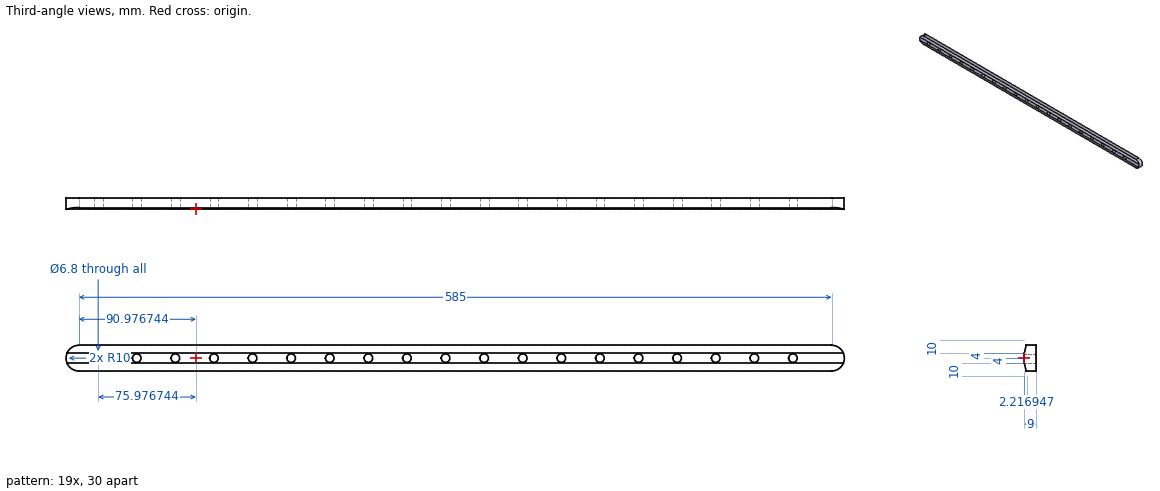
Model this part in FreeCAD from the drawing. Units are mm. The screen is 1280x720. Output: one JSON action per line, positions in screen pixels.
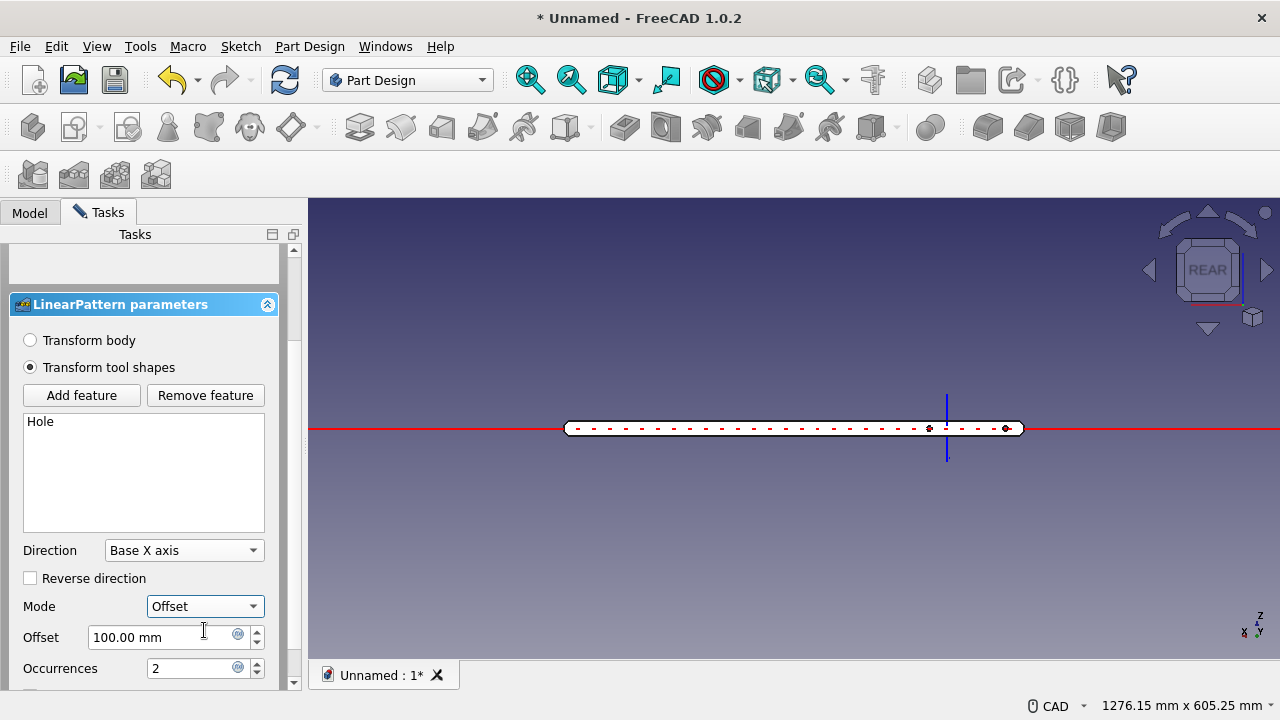
{"action": "triple_click", "coordinate": [170, 638]}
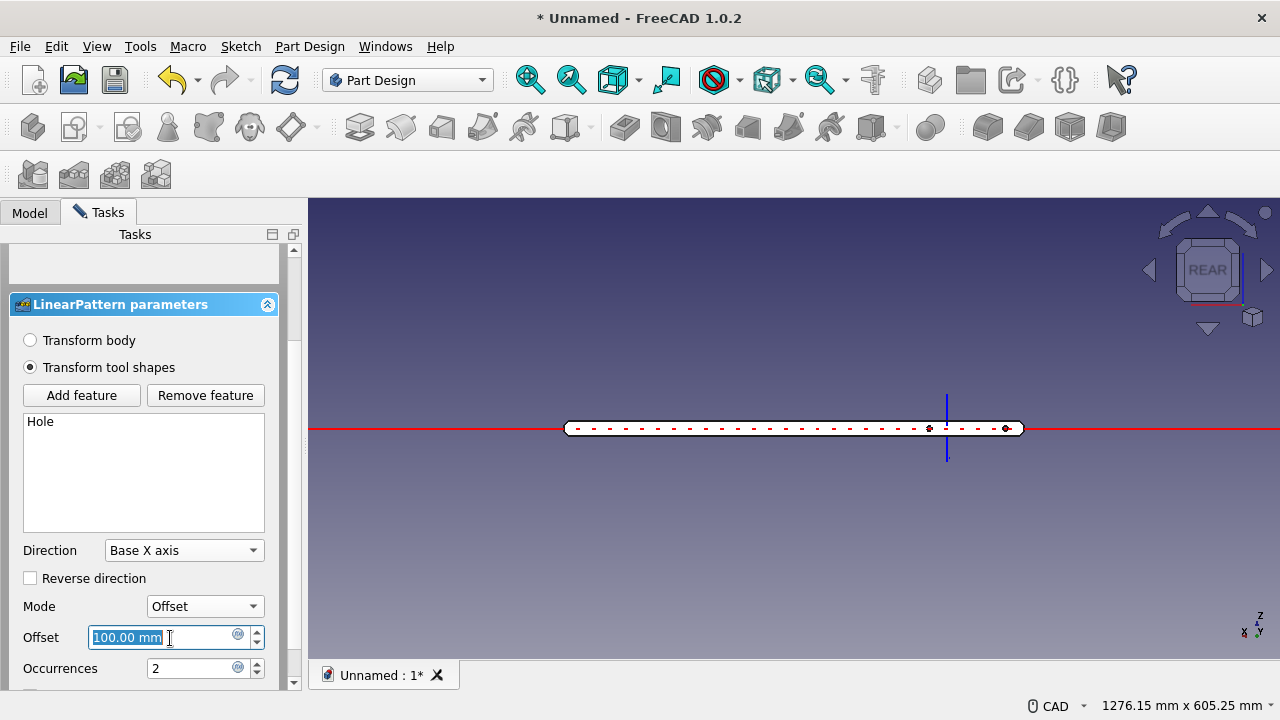
{"action": "type", "text": "30"}
{"action": "key", "text": "Tab"}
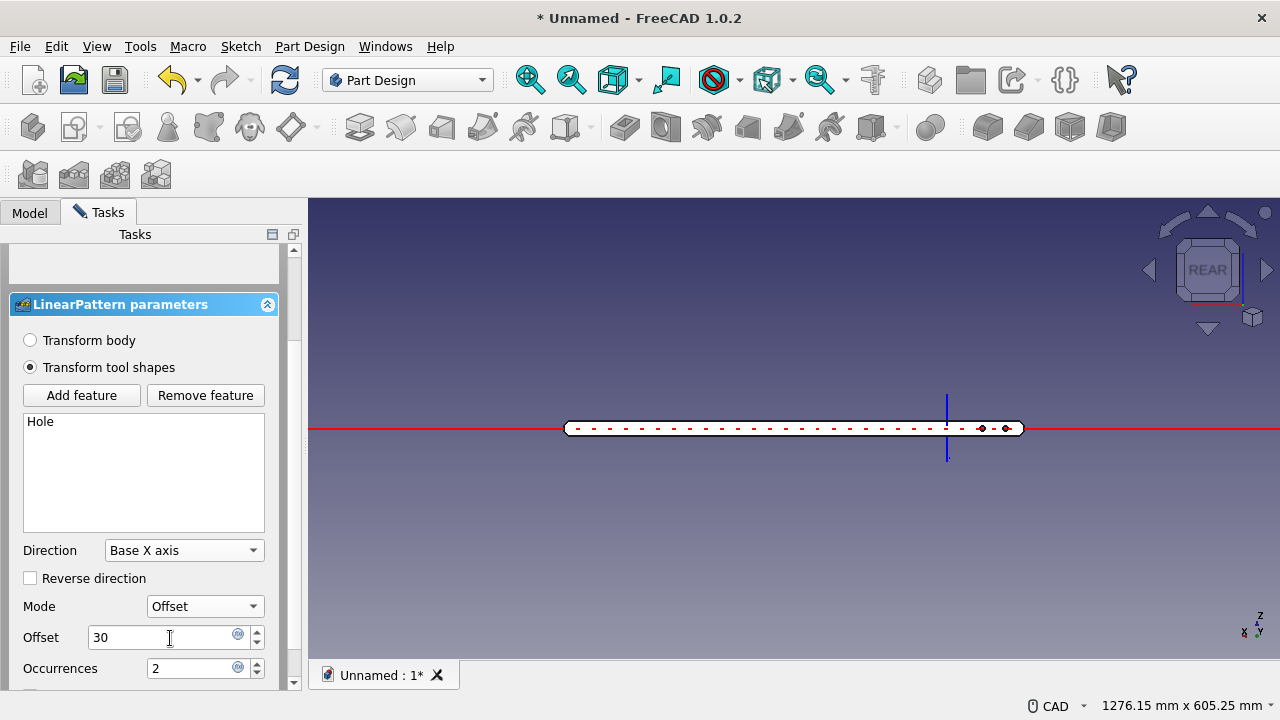
{"action": "triple_click", "coordinate": [199, 668]}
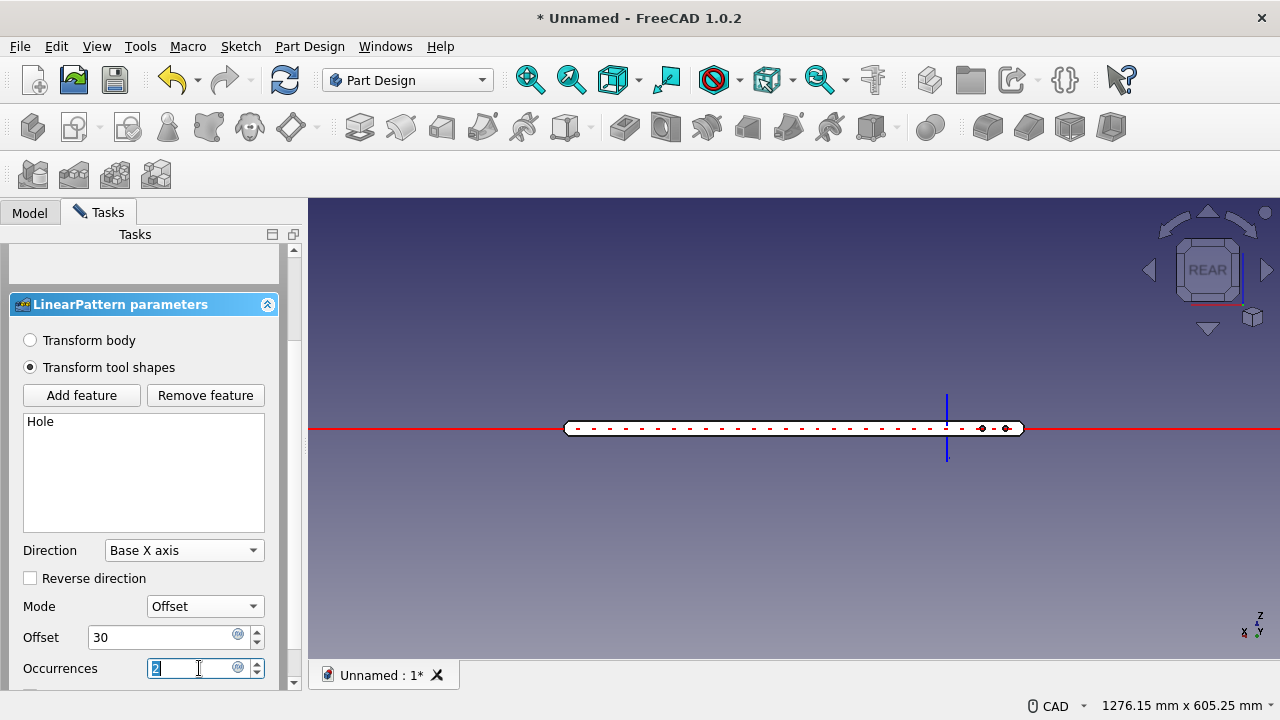
{"action": "type", "text": "19"}
{"action": "key", "text": "Tab"}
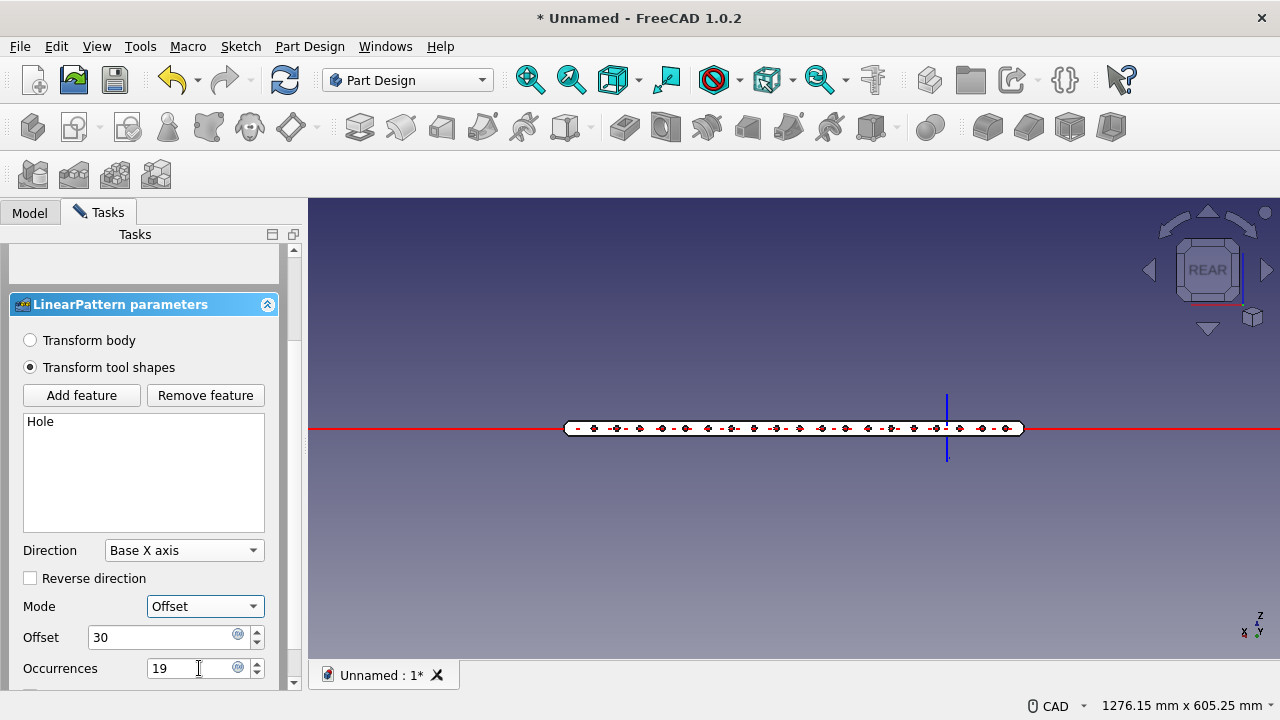
{"action": "scroll", "coordinate": [294, 467], "scroll_direction": "up", "scroll_amount": 3}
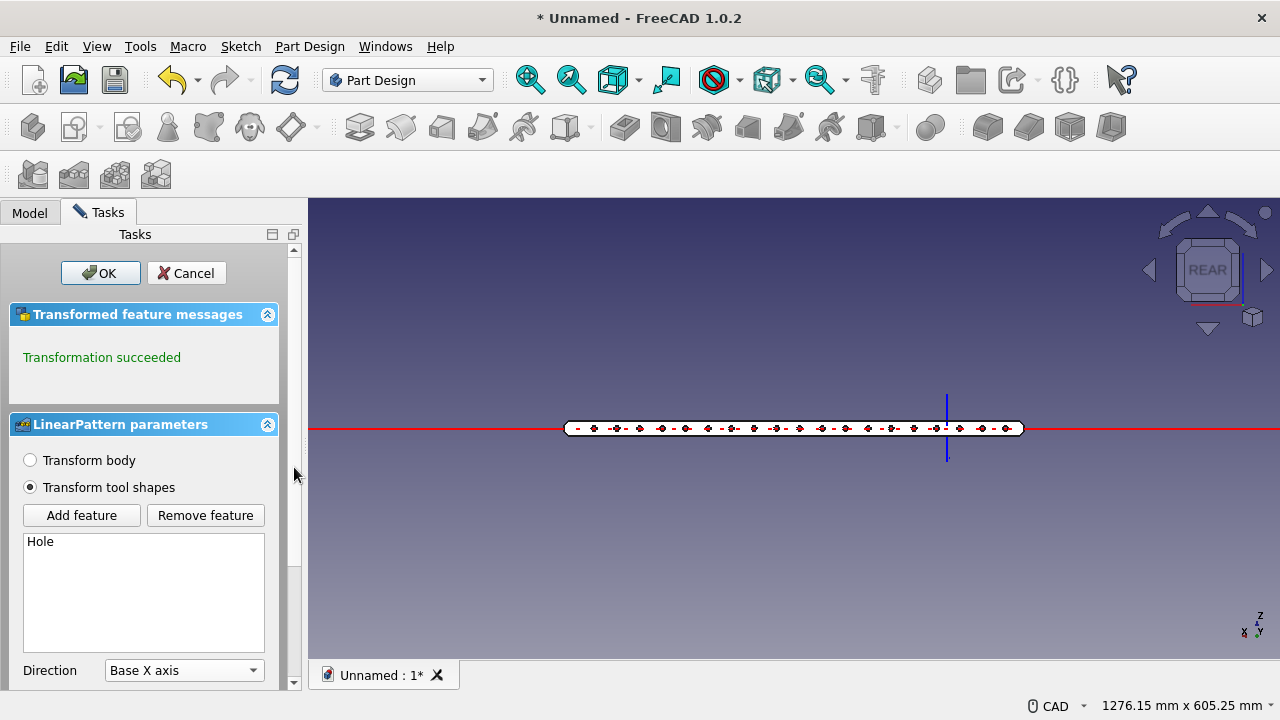
{"action": "left_click", "coordinate": [101, 273]}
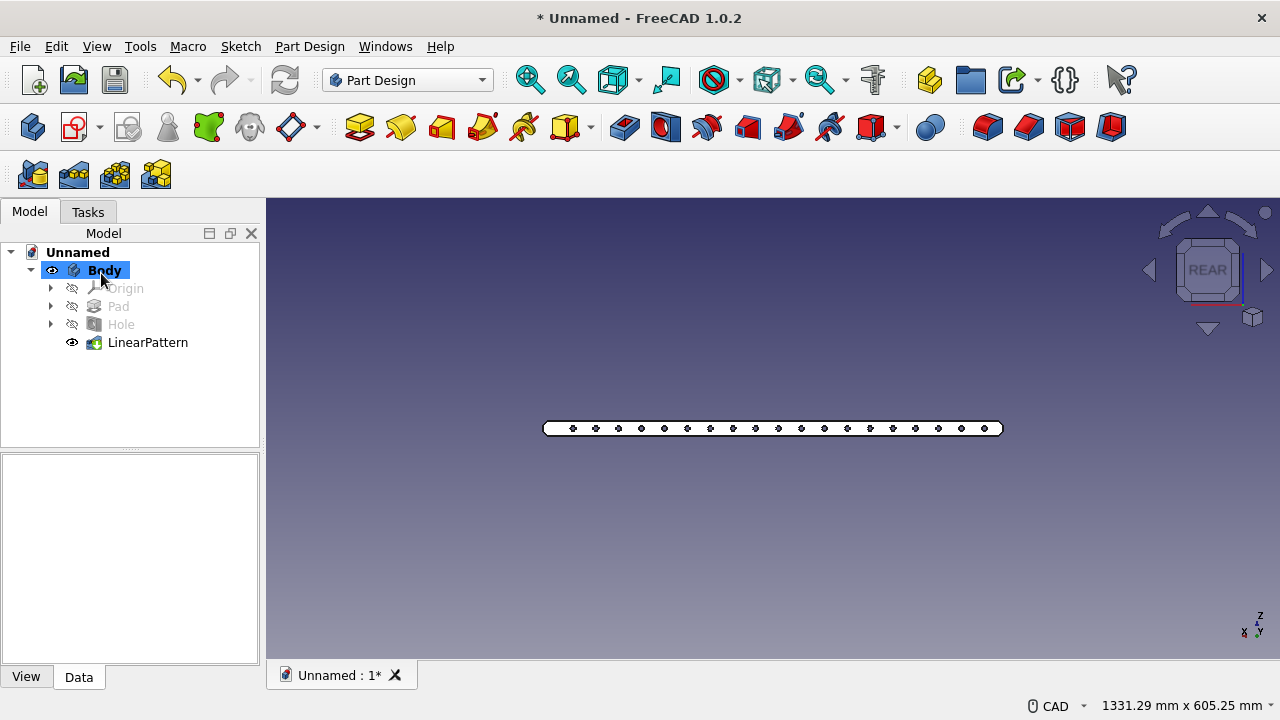
{"action": "left_click", "coordinate": [51, 288]}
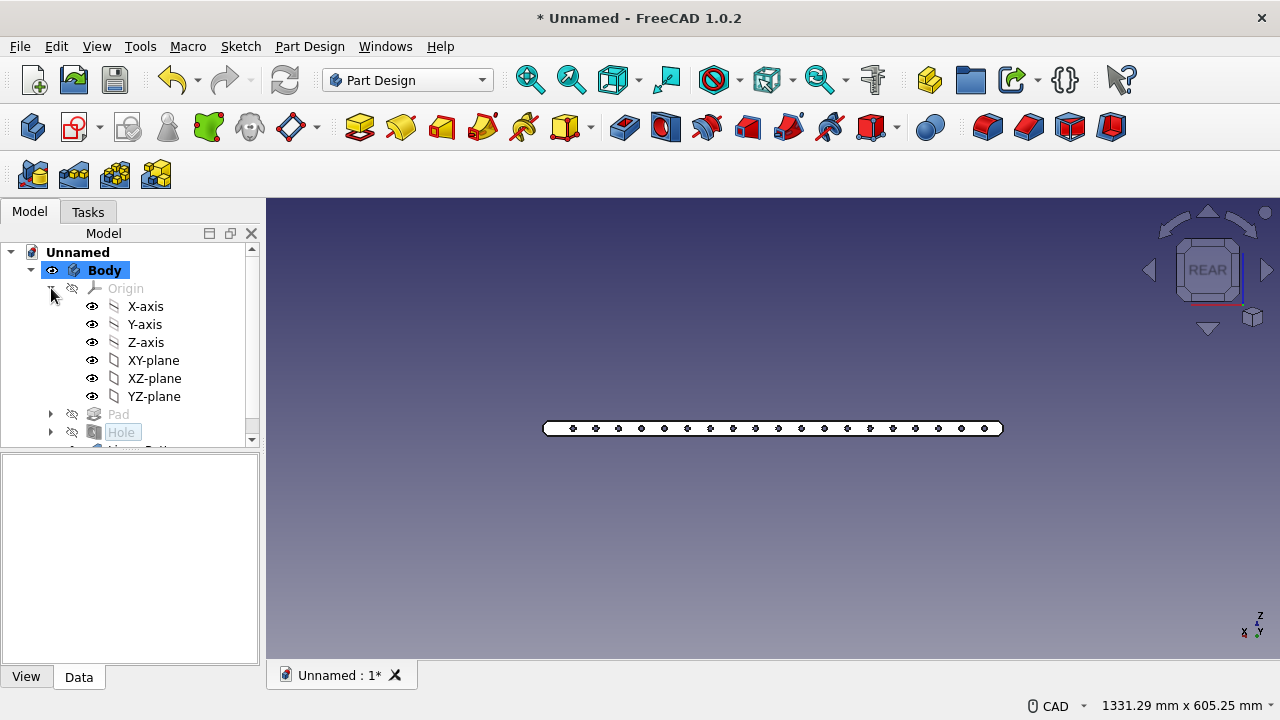
{"action": "left_click", "coordinate": [137, 396]}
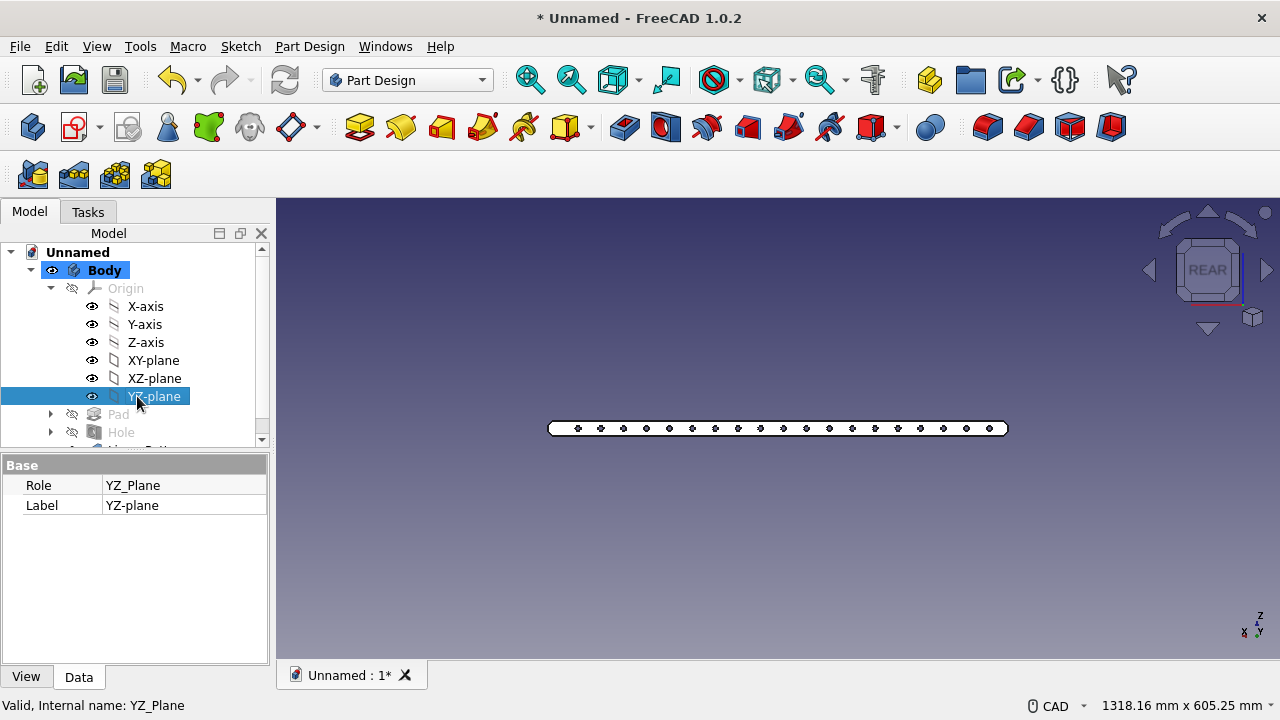
{"action": "left_click", "coordinate": [290, 128]}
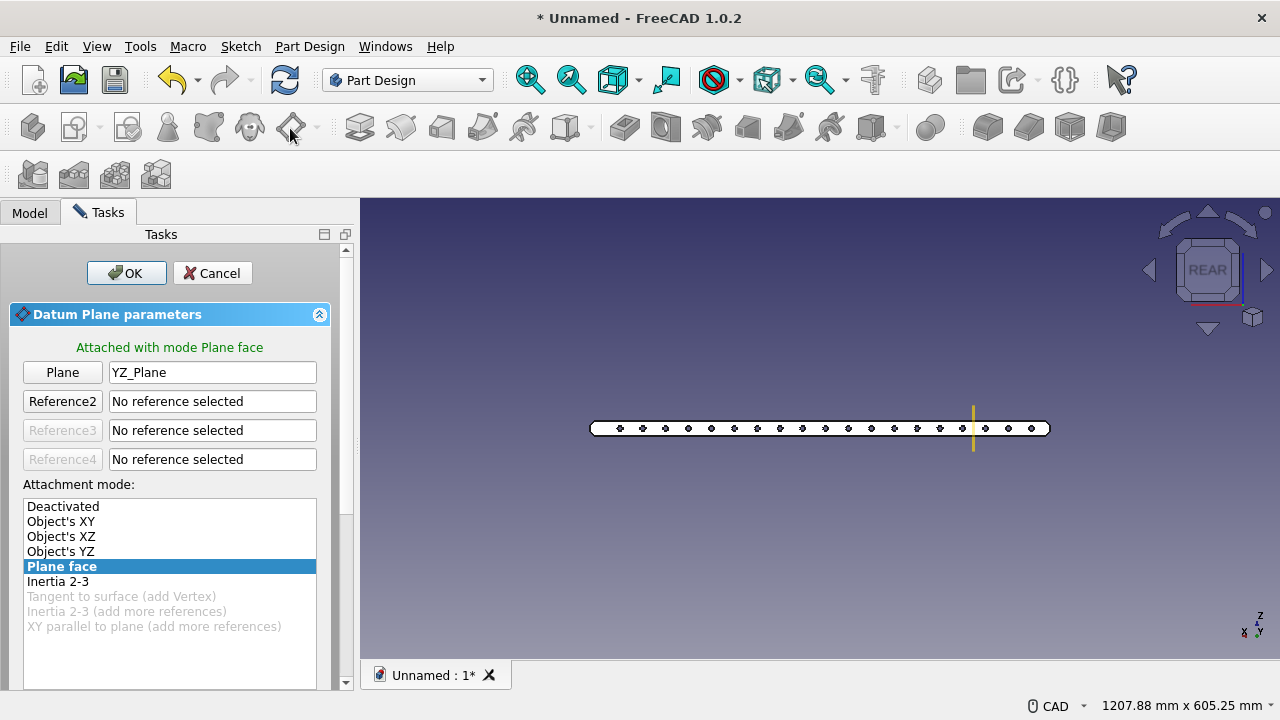
{"action": "scroll", "coordinate": [346, 467], "scroll_direction": "down", "scroll_amount": 4}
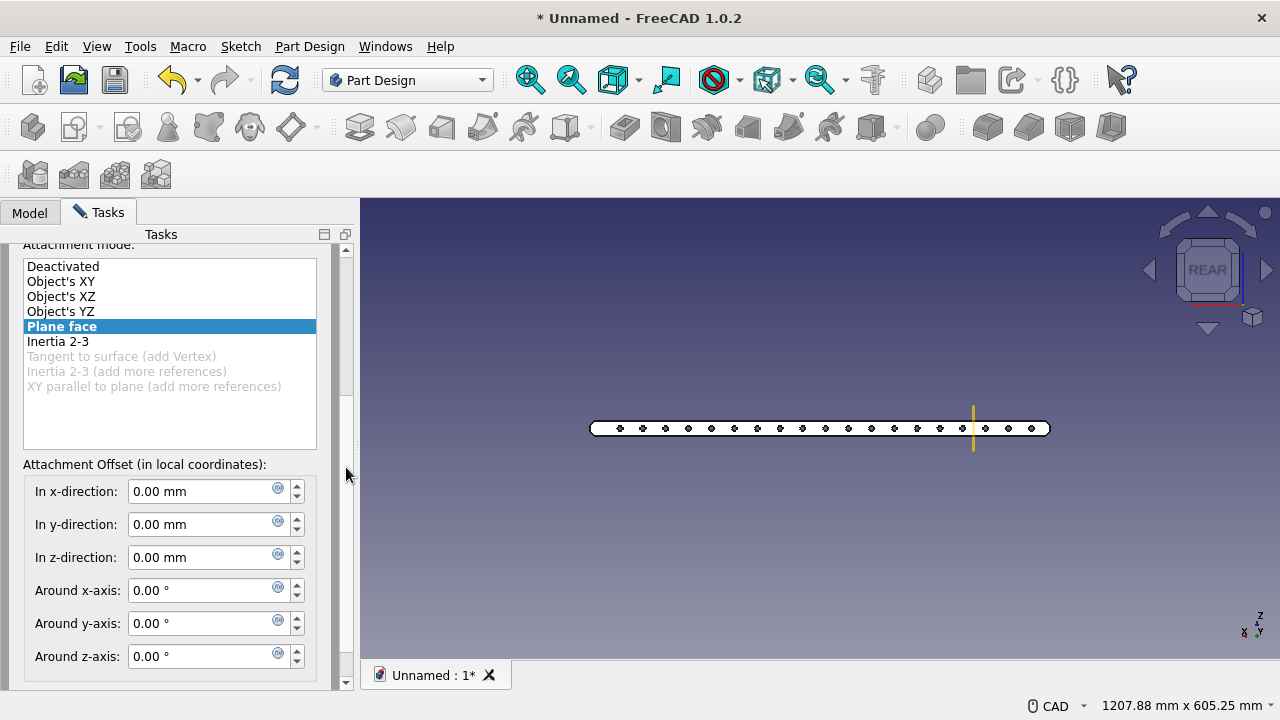
{"action": "triple_click", "coordinate": [210, 558]}